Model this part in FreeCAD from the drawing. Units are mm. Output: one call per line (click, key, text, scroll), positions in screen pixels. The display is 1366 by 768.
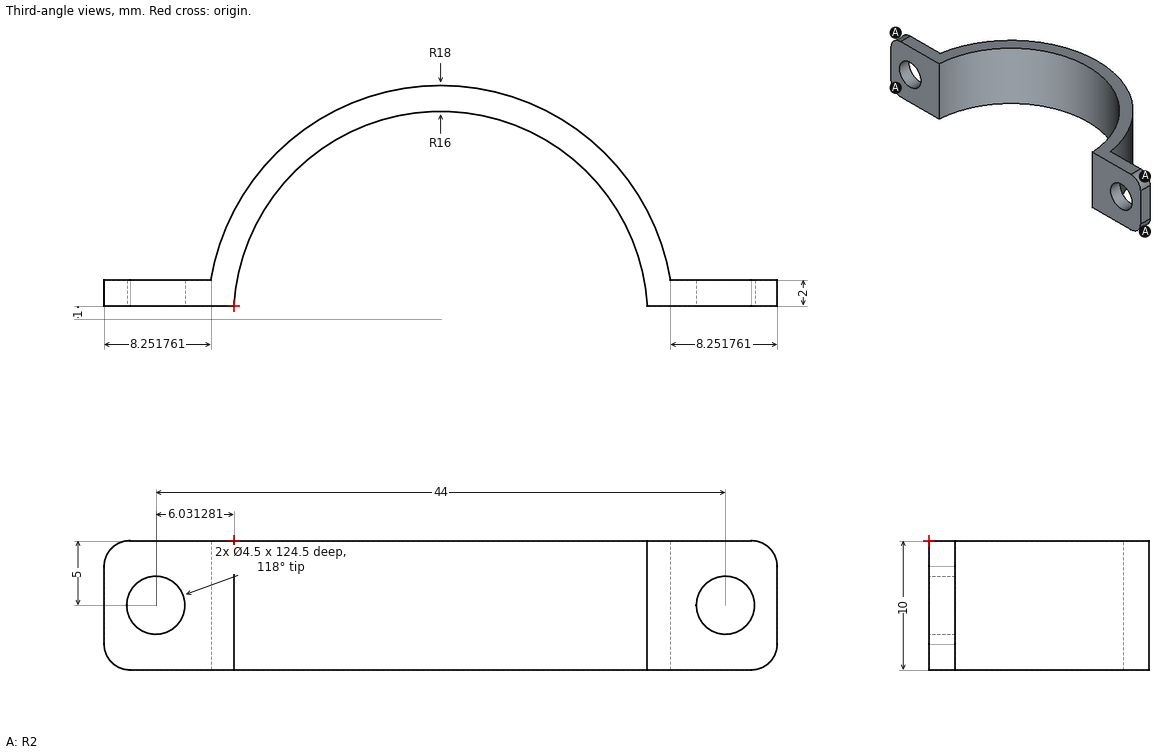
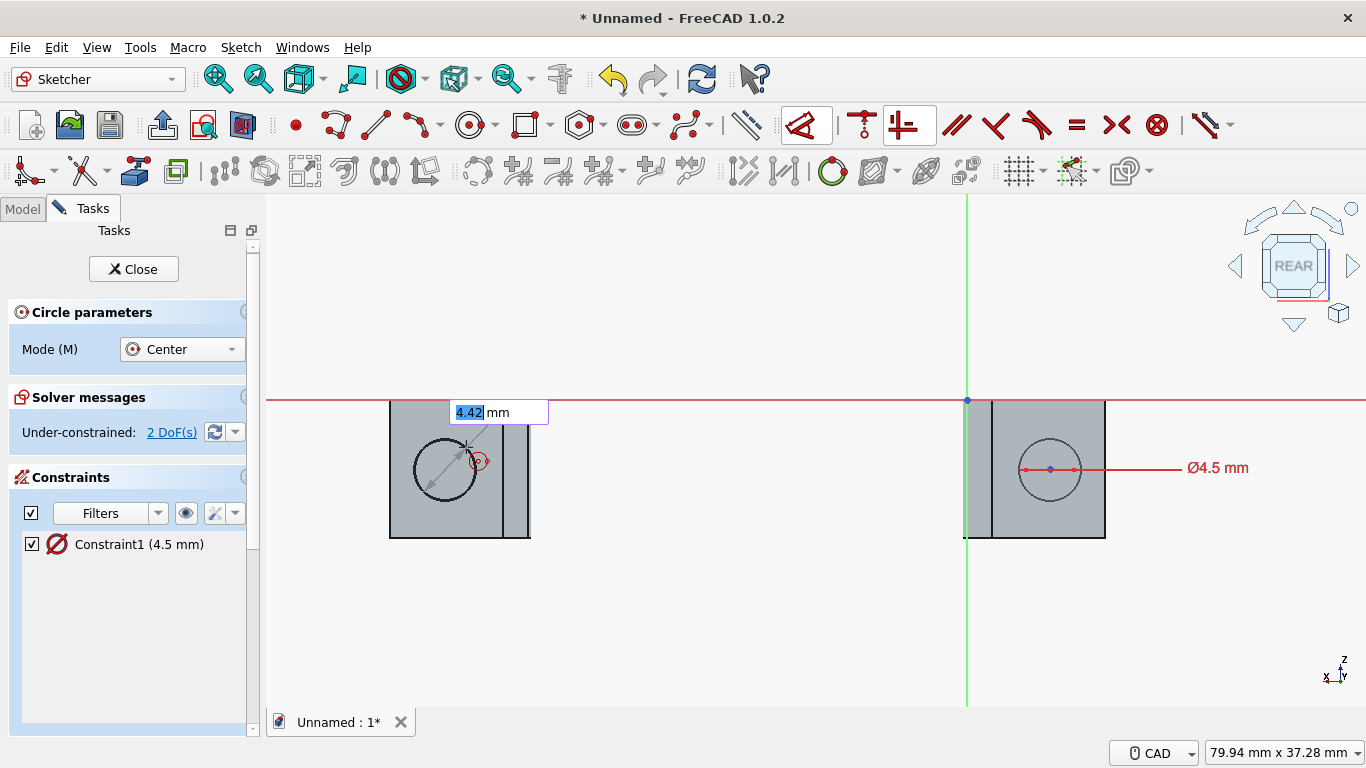
text(4.5)
key(Return)
key(Escape)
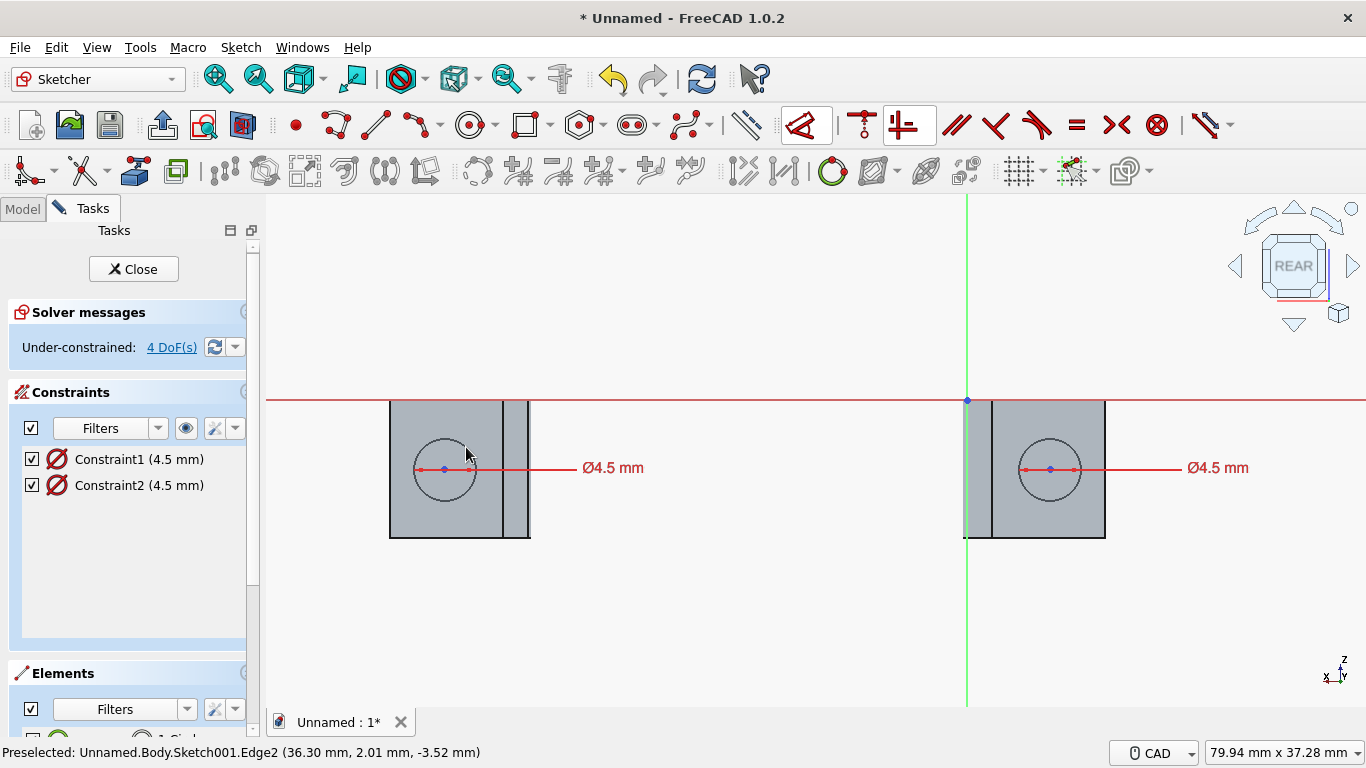
click(1050, 470)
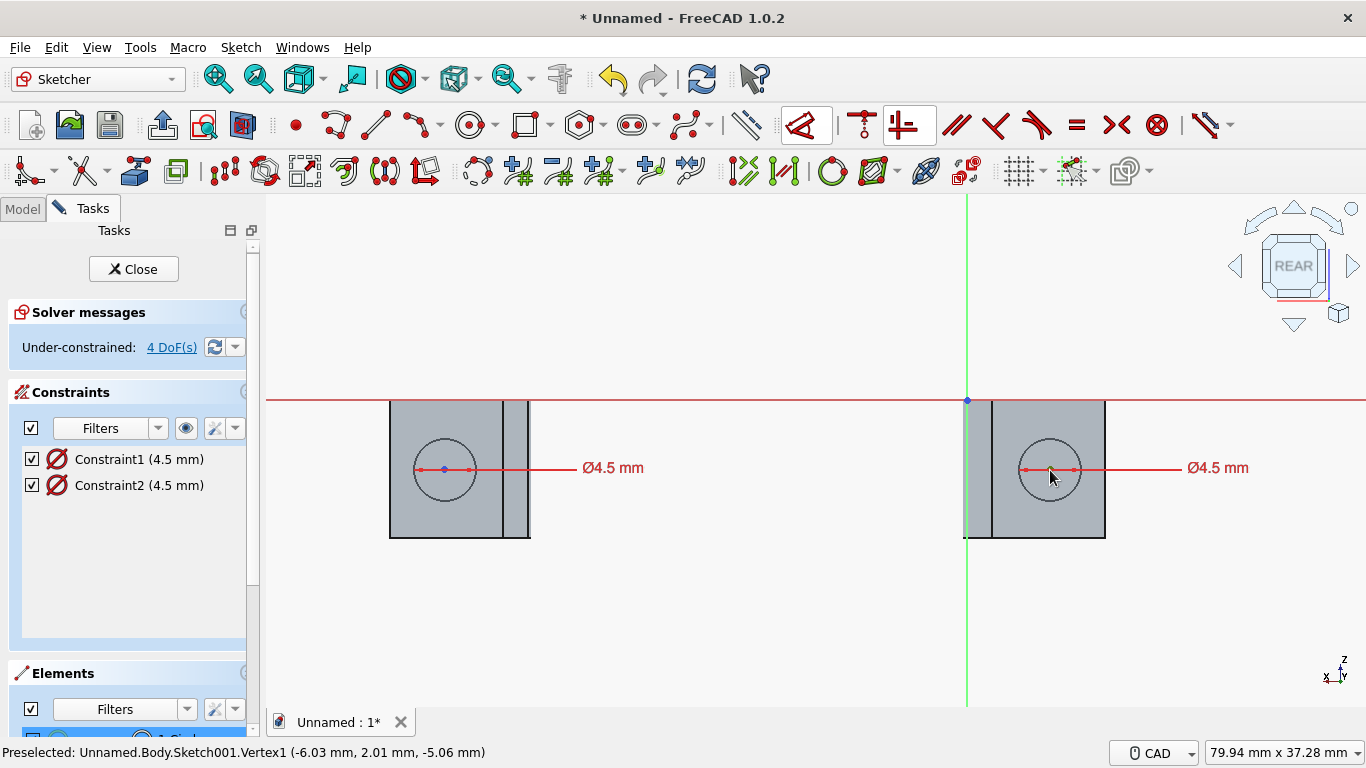
key(i)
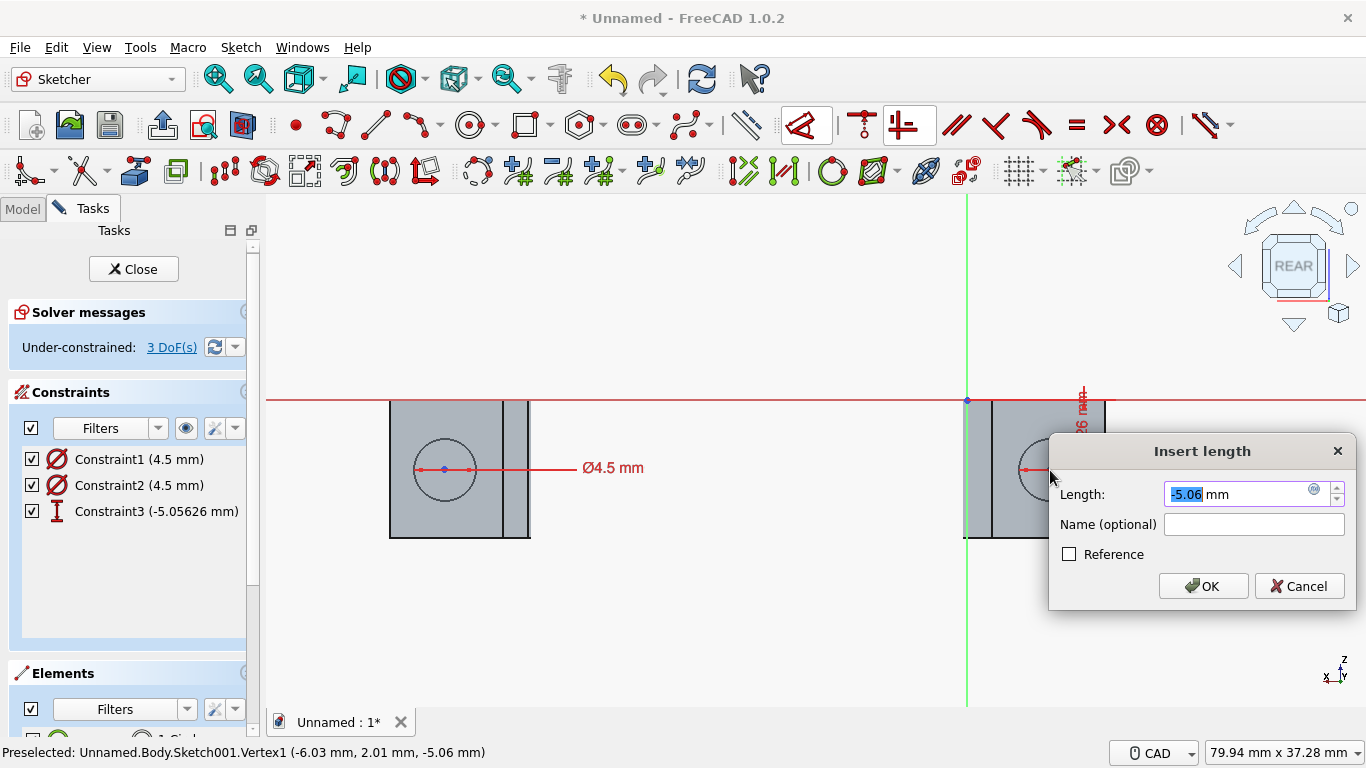
text(-5)
key(Return)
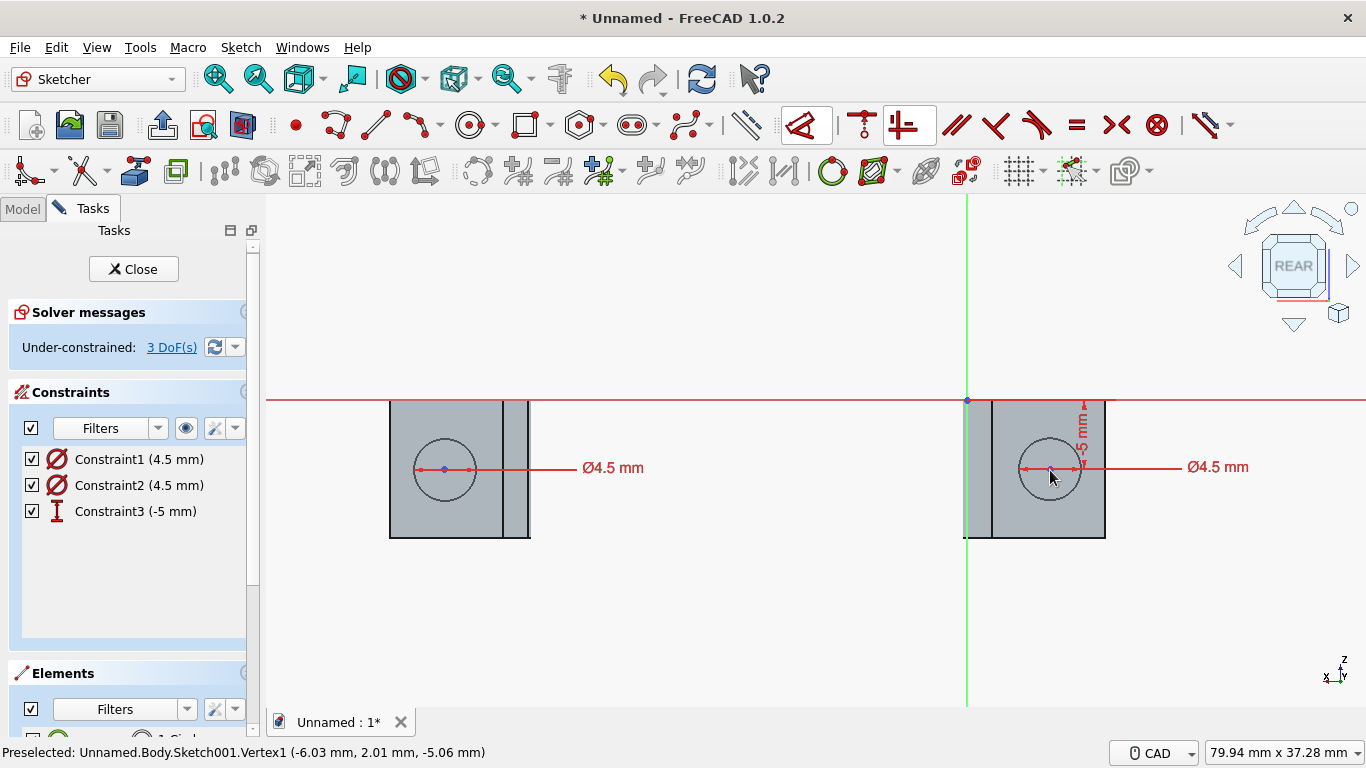
click(445, 470)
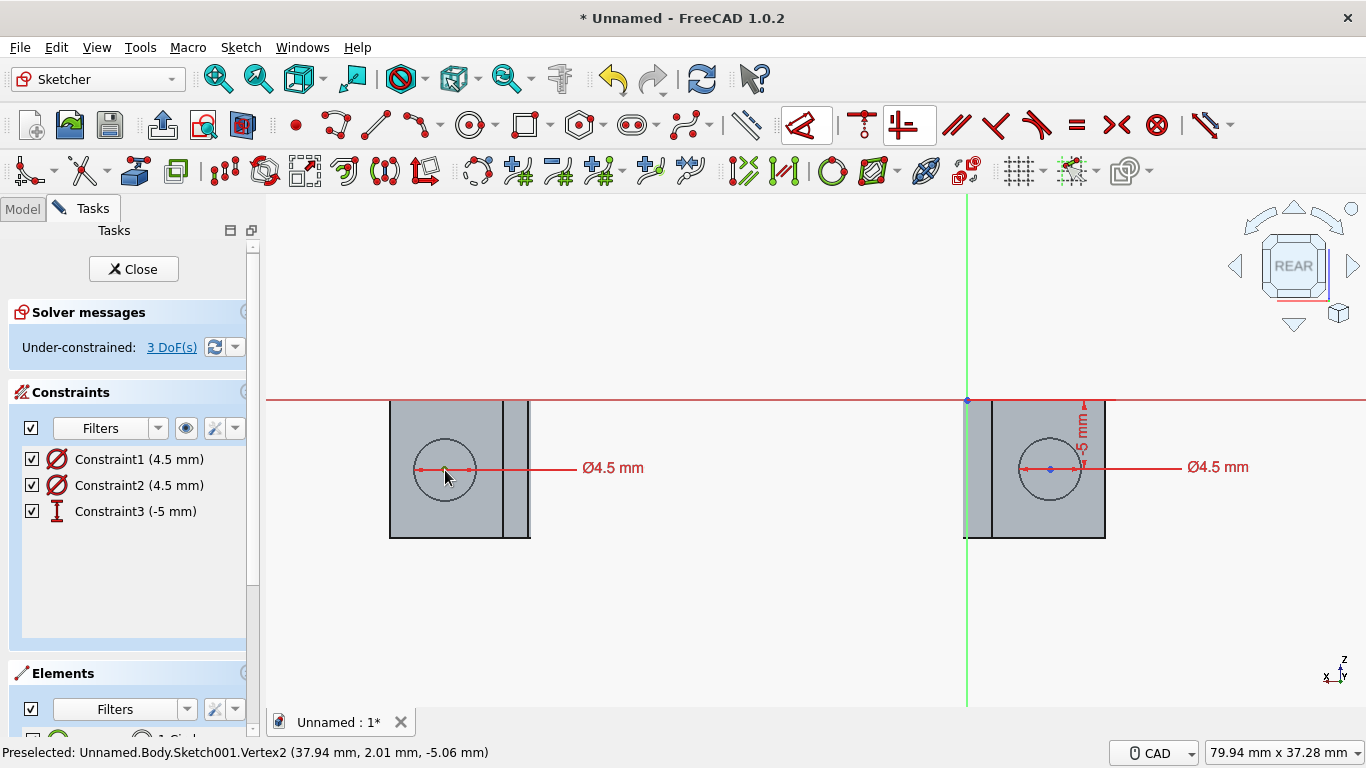
click(826, 126)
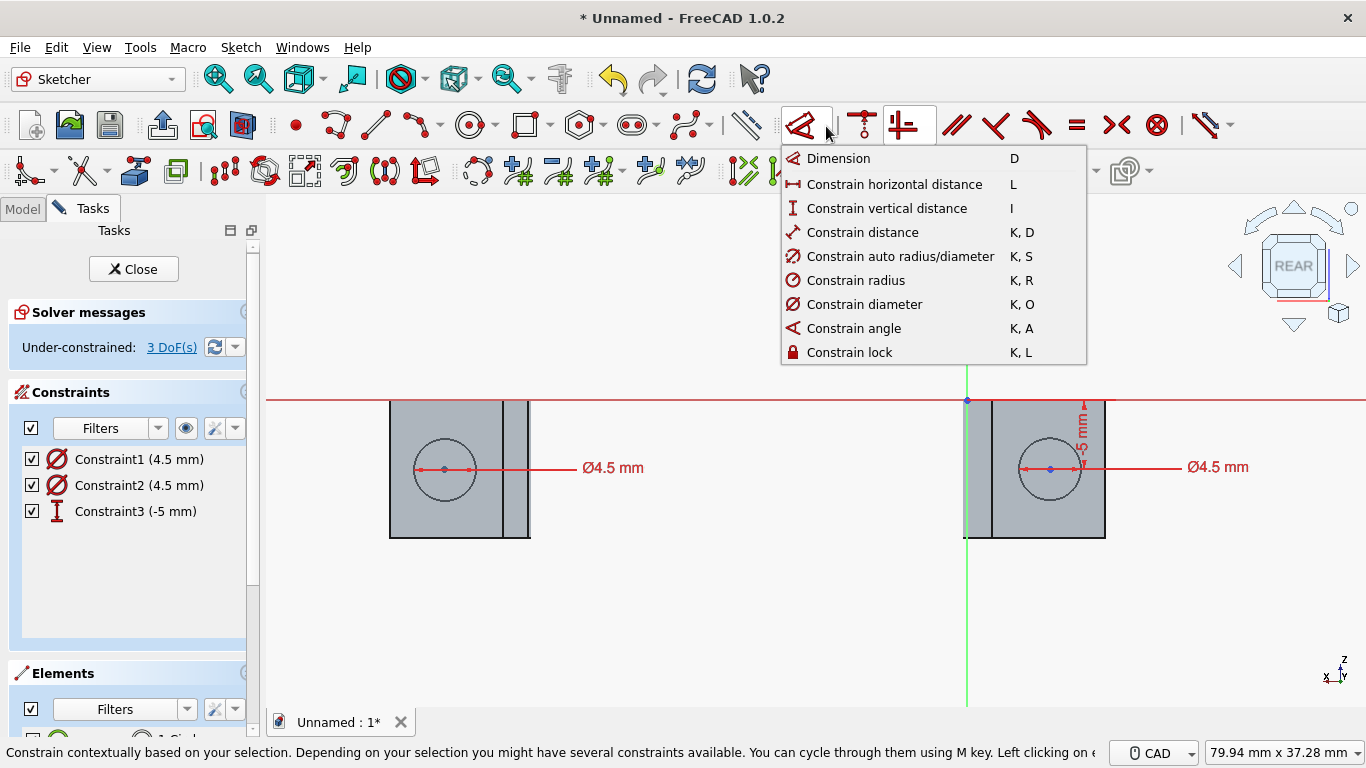
click(934, 208)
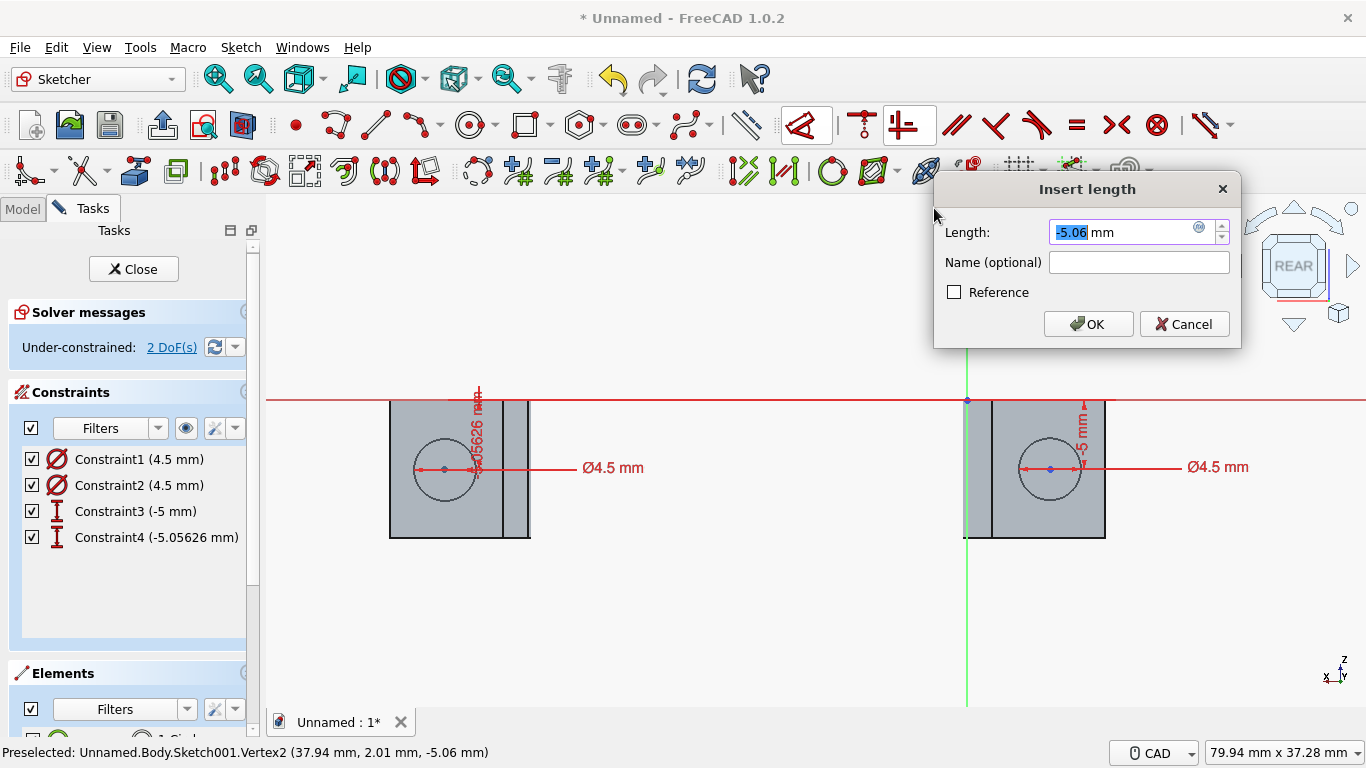
text(-5)
key(Return)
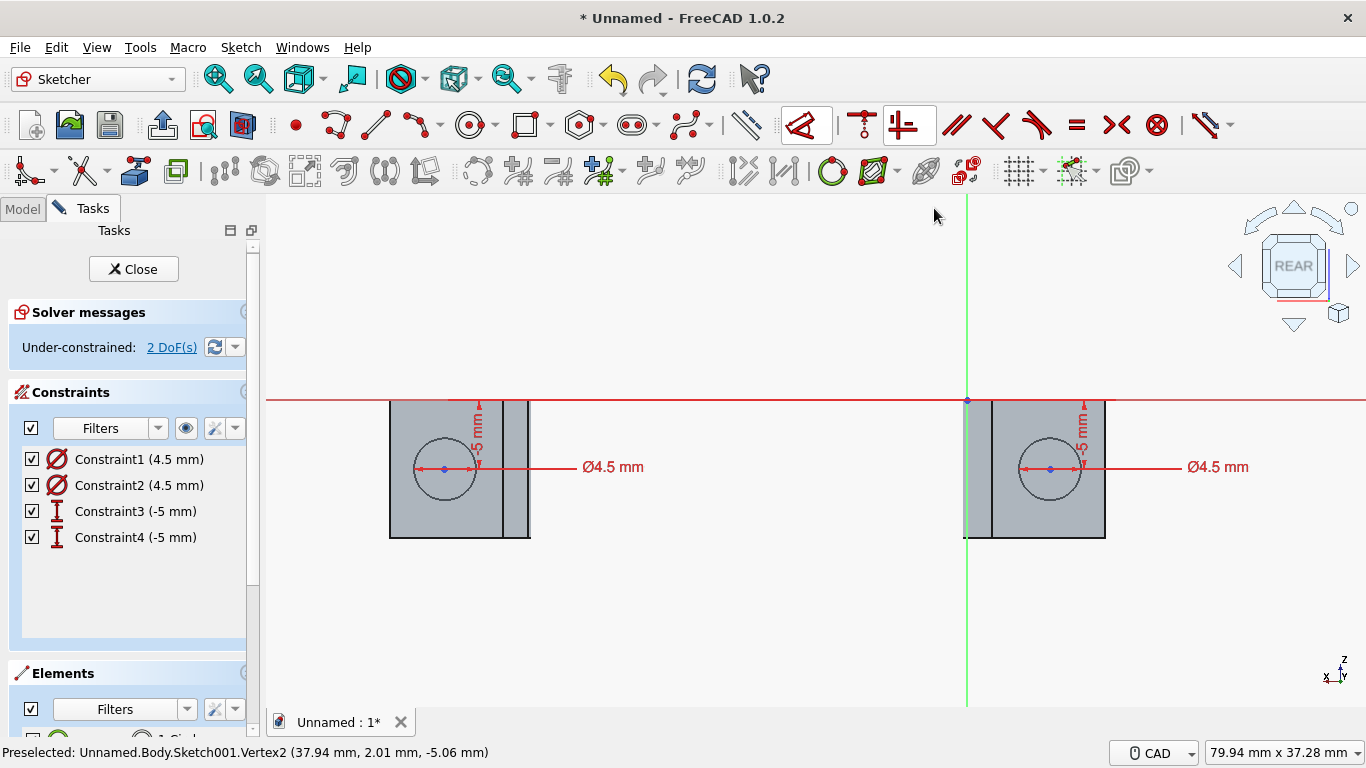
click(1050, 469)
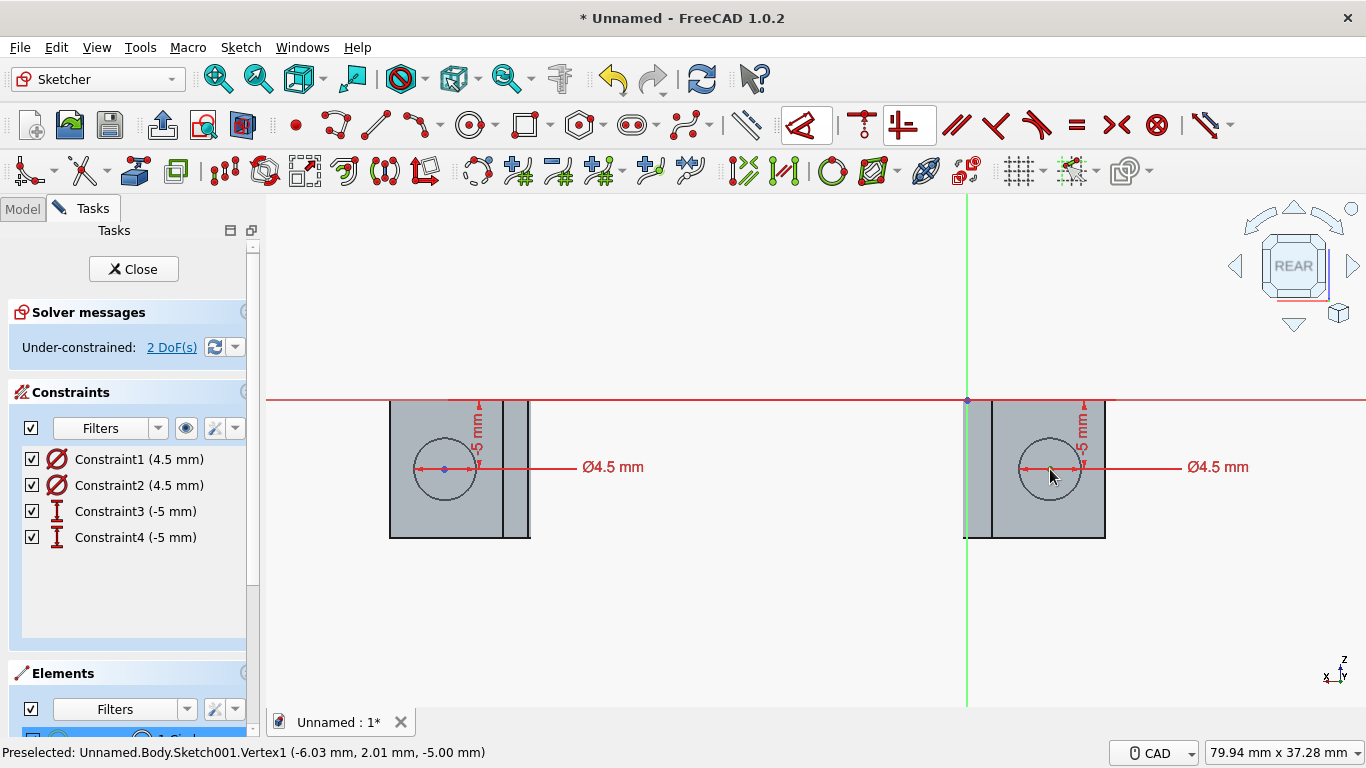
click(445, 469)